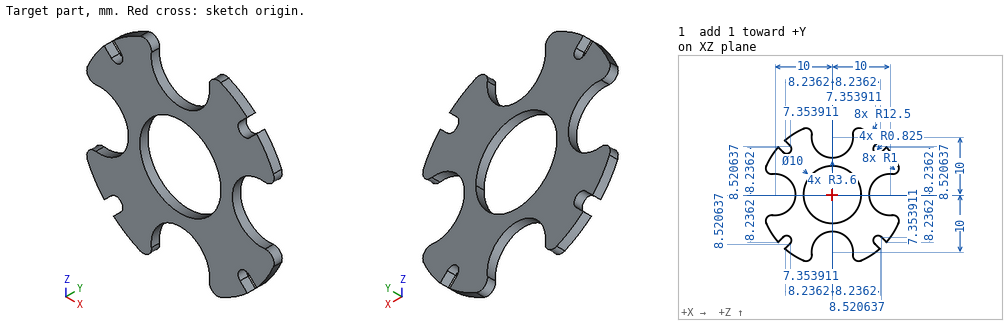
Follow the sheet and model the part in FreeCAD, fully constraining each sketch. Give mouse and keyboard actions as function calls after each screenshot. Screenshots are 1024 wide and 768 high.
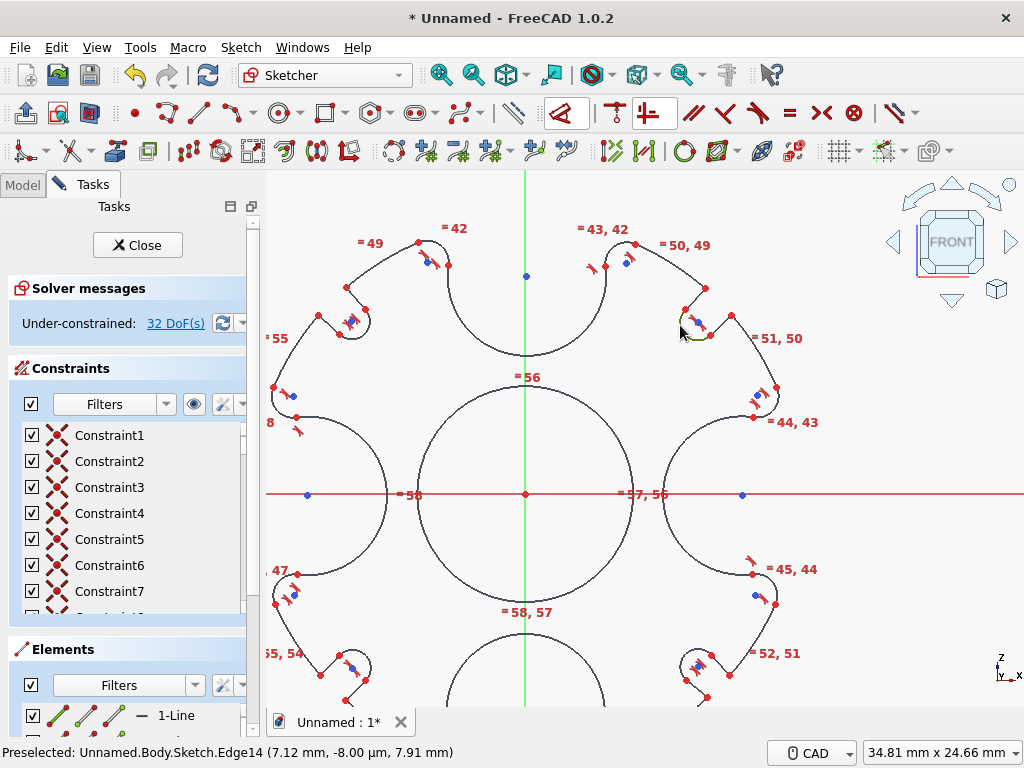
click(696, 649)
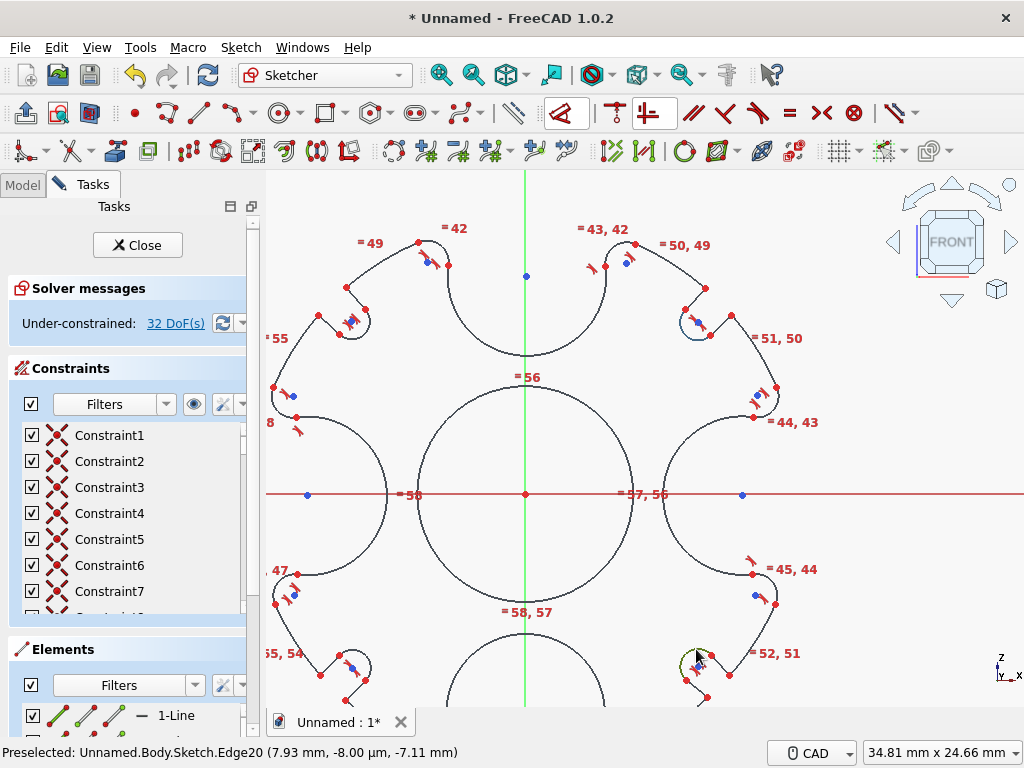
click(371, 665)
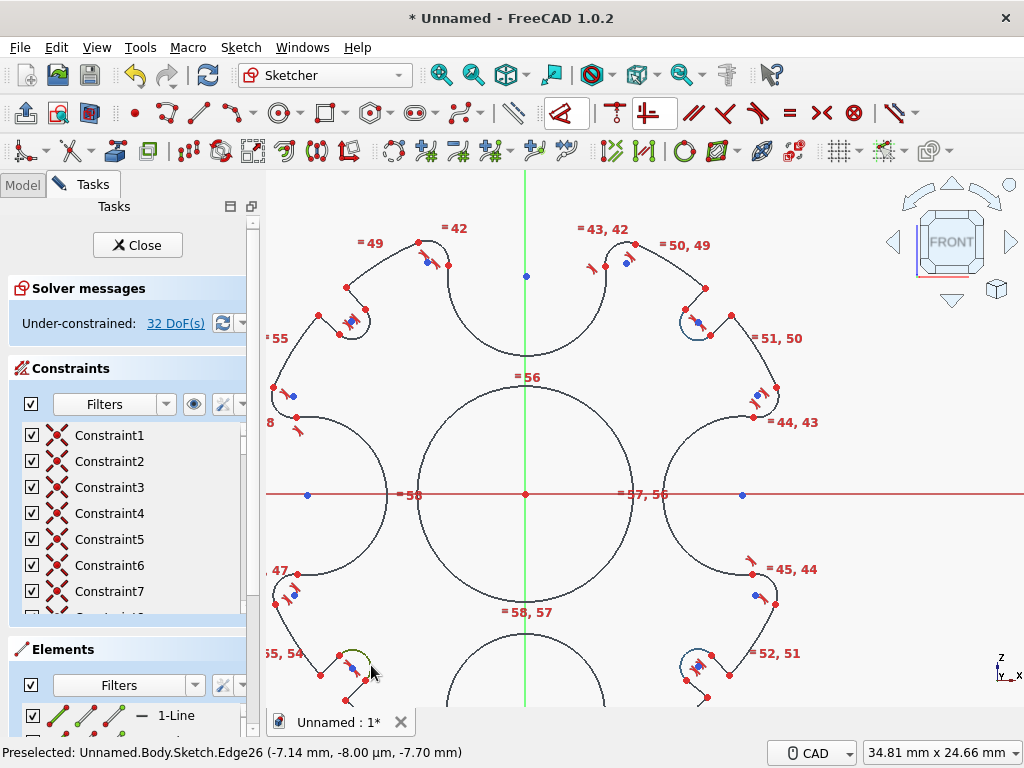
click(355, 339)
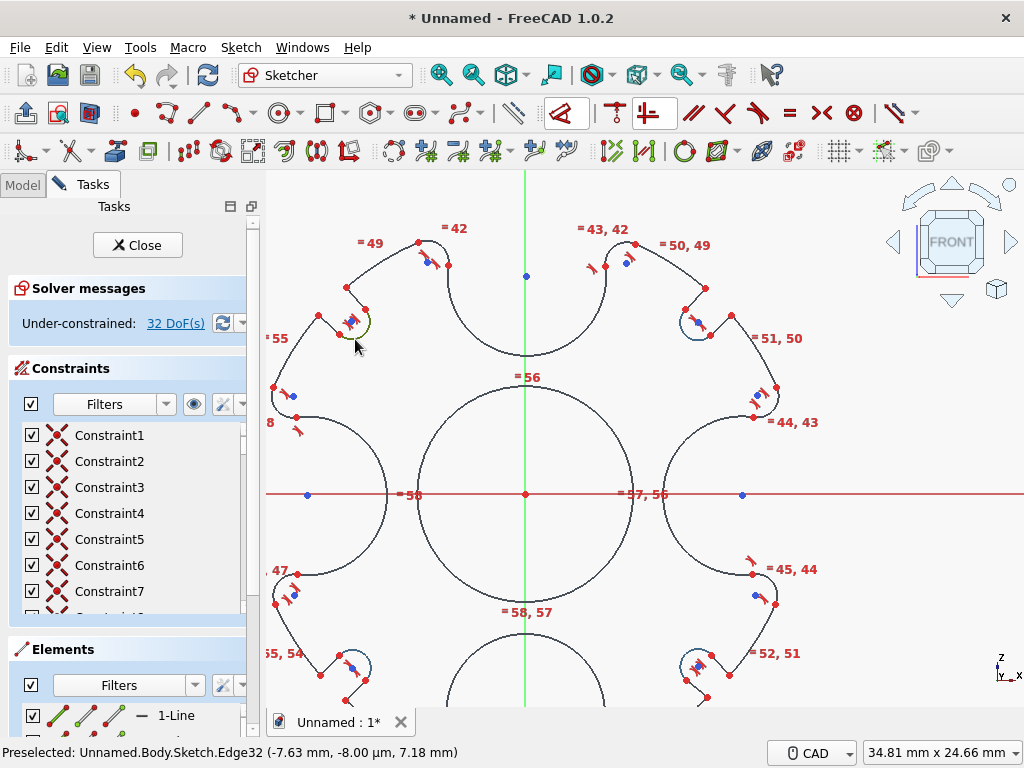
click(790, 114)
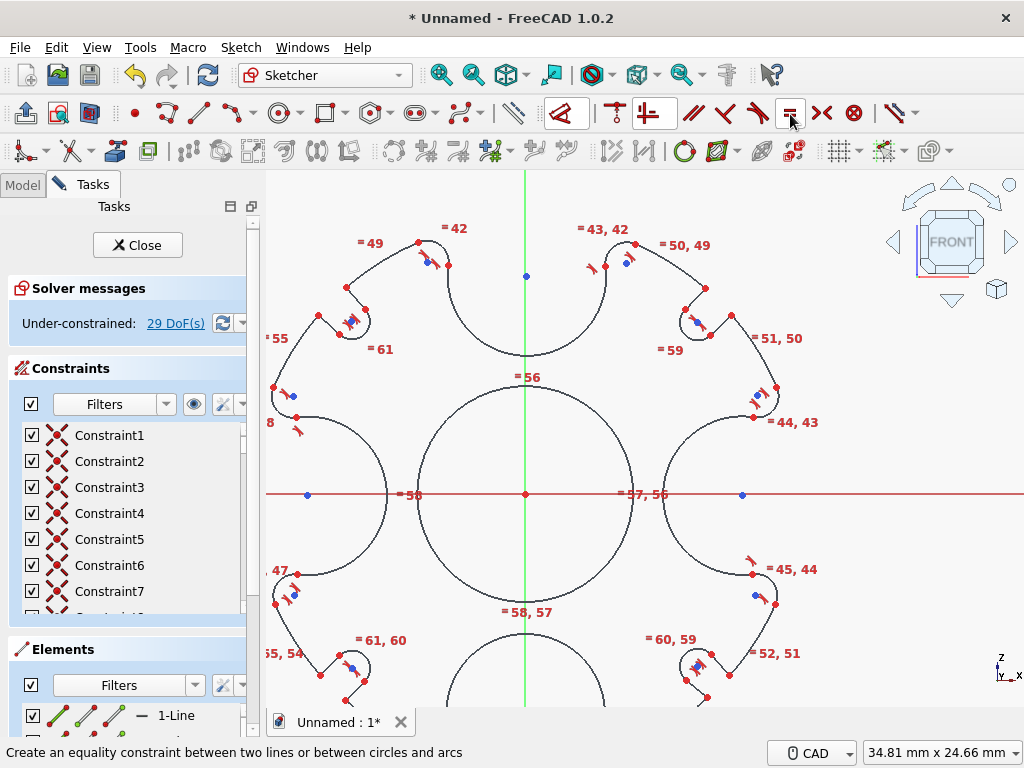
click(527, 277)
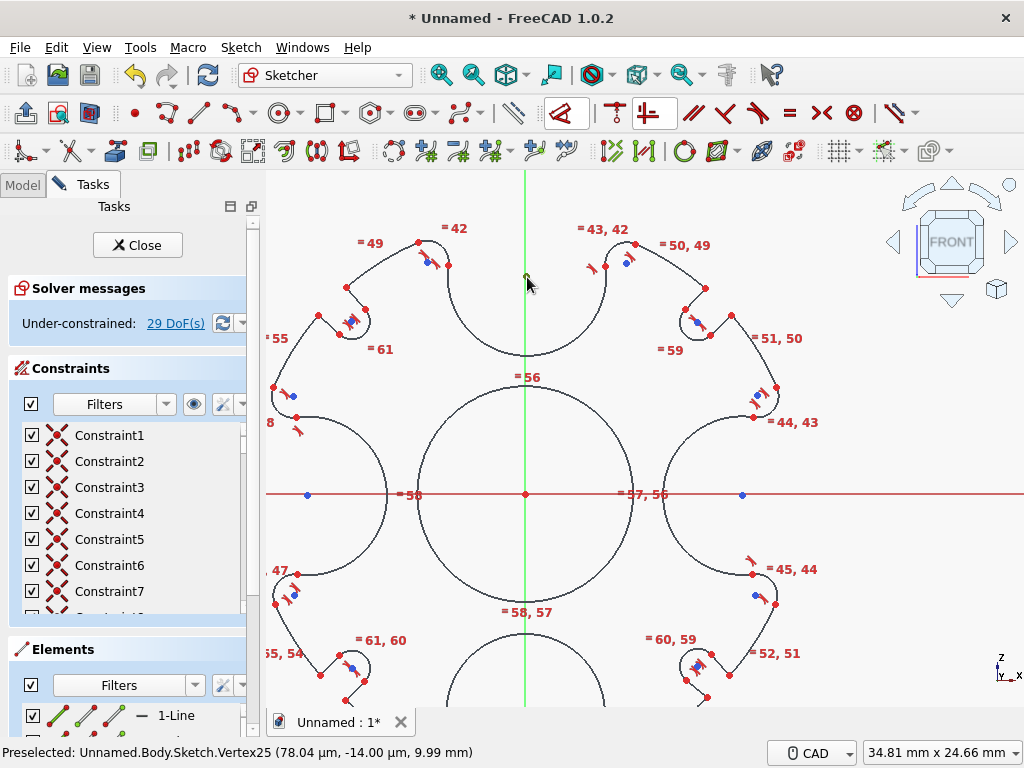
click(525, 542)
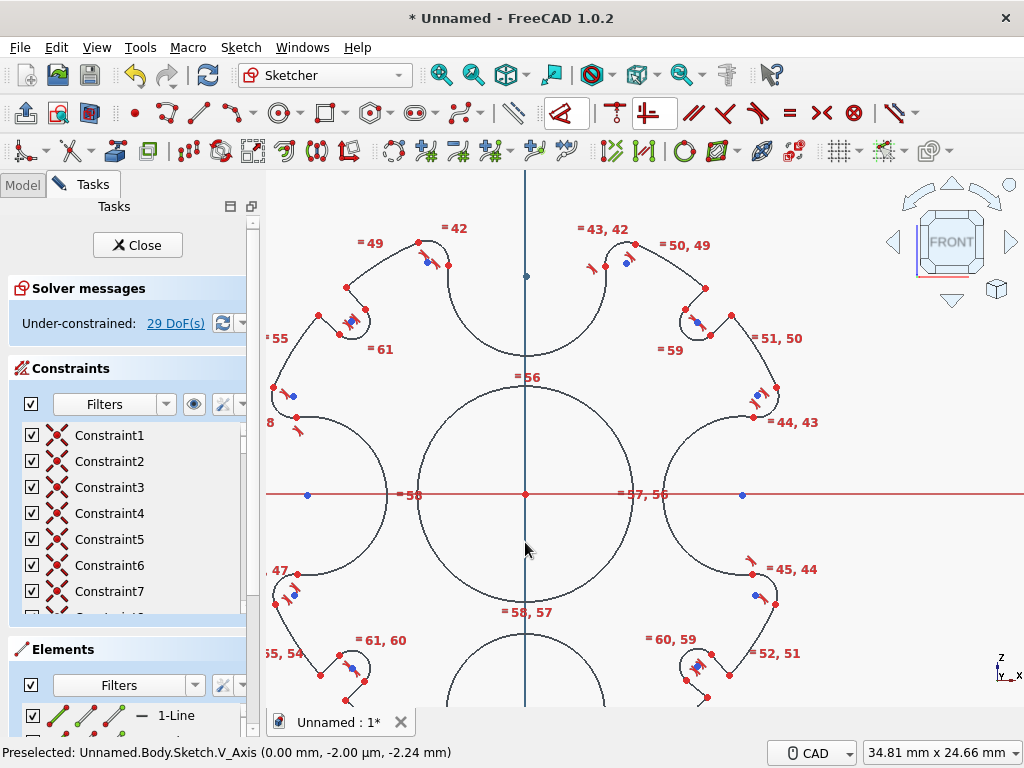
click(616, 114)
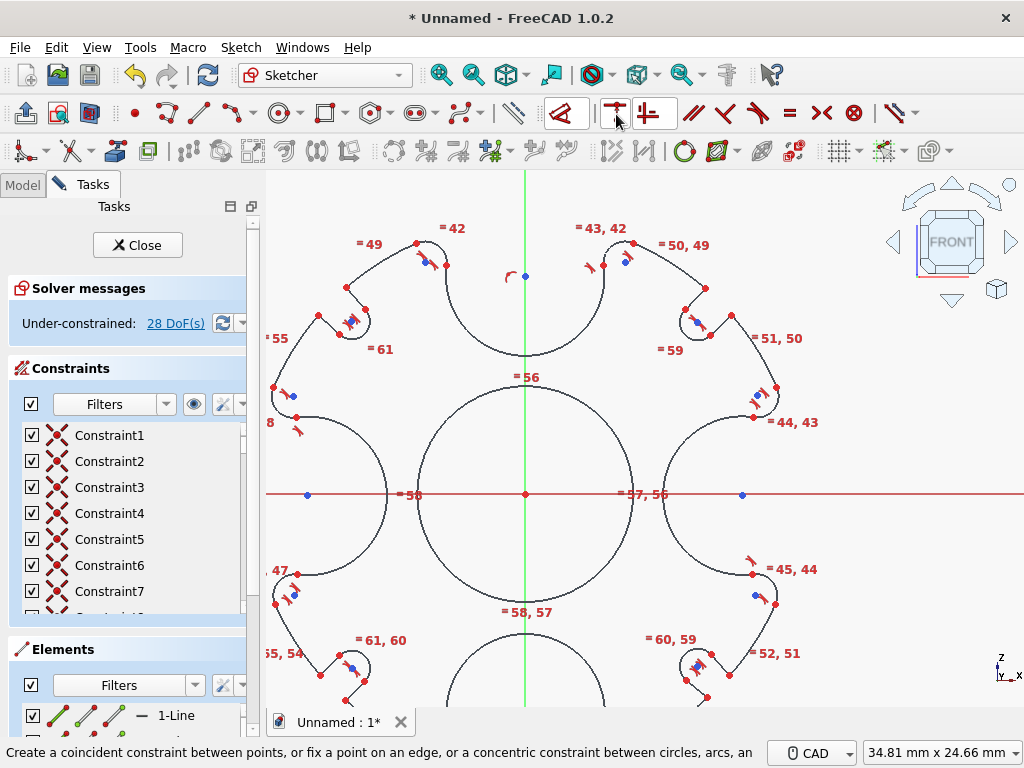
click(742, 496)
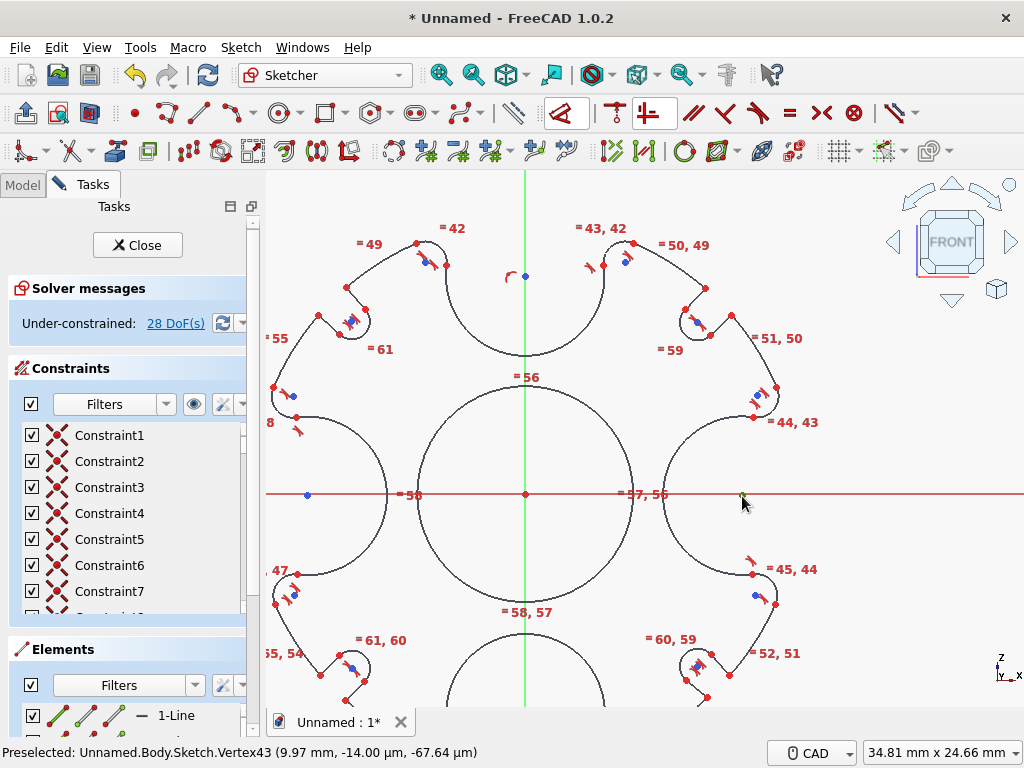
click(334, 494)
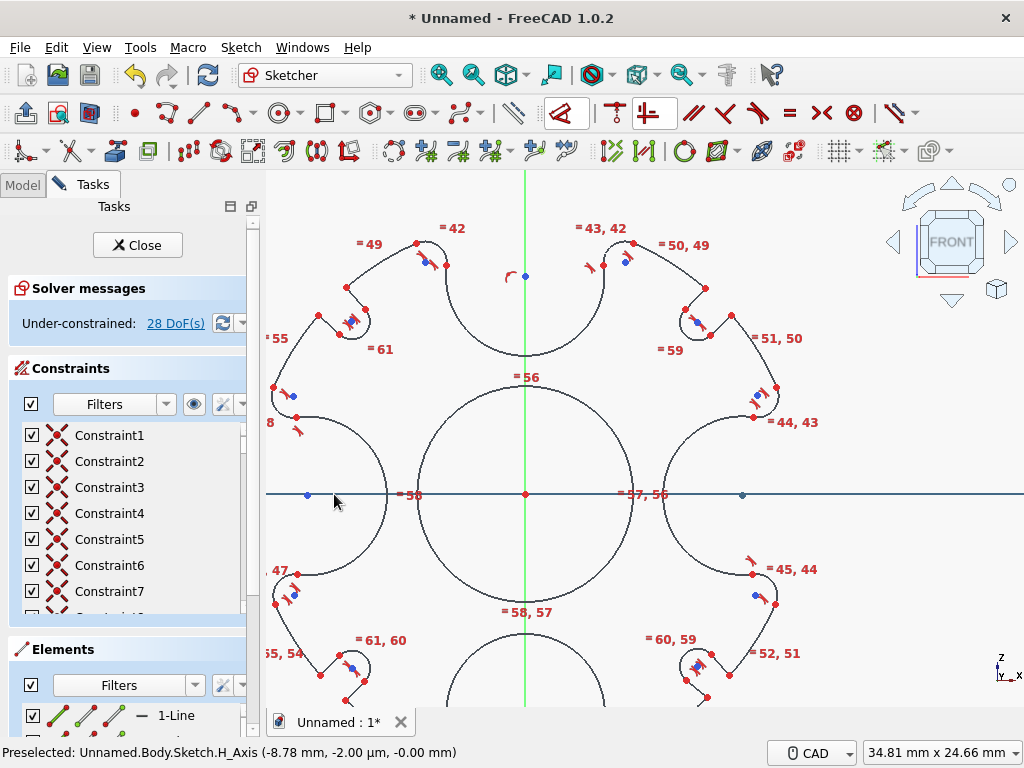
key(c)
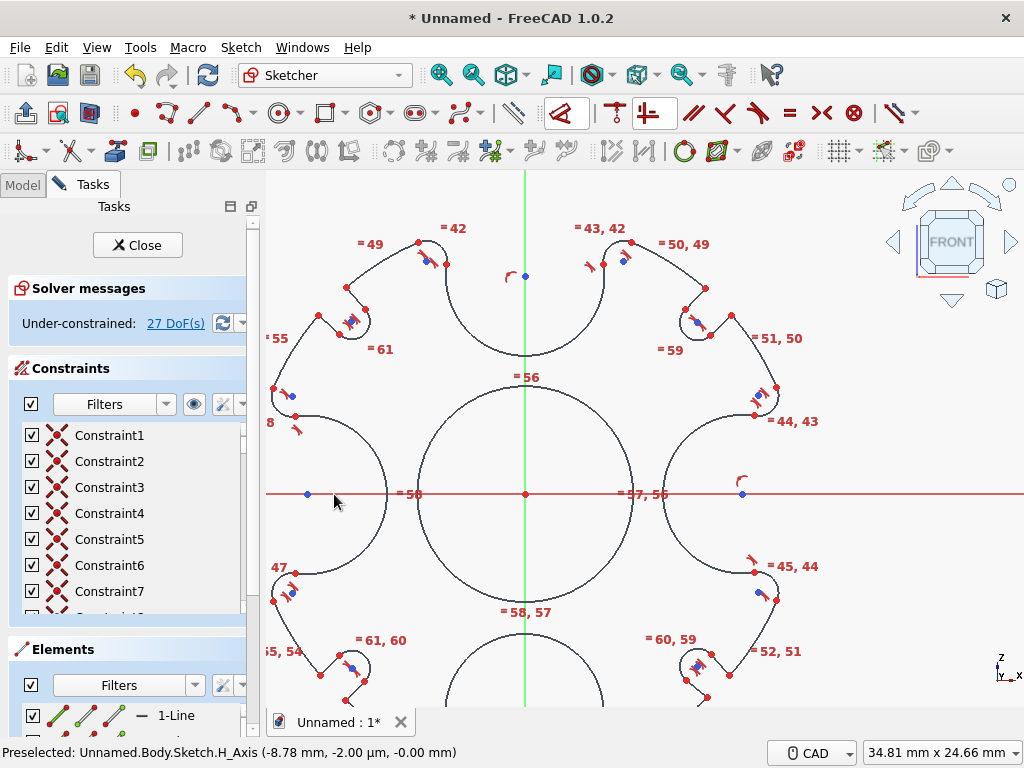
scroll(681, 325, down, 2)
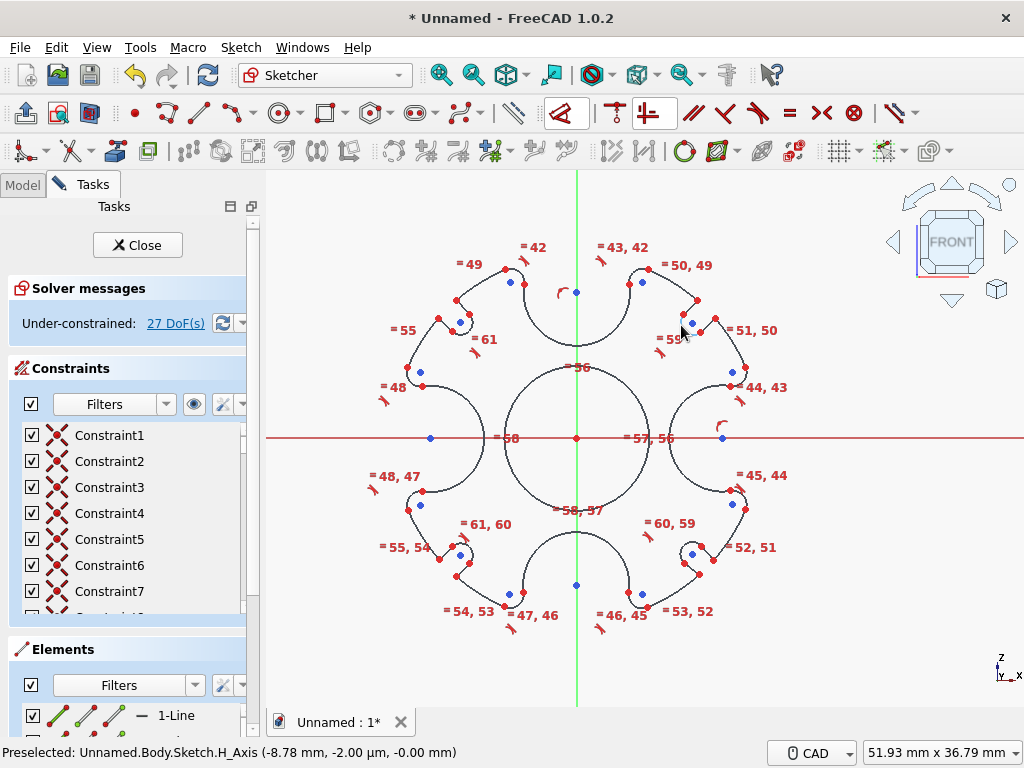
click(576, 585)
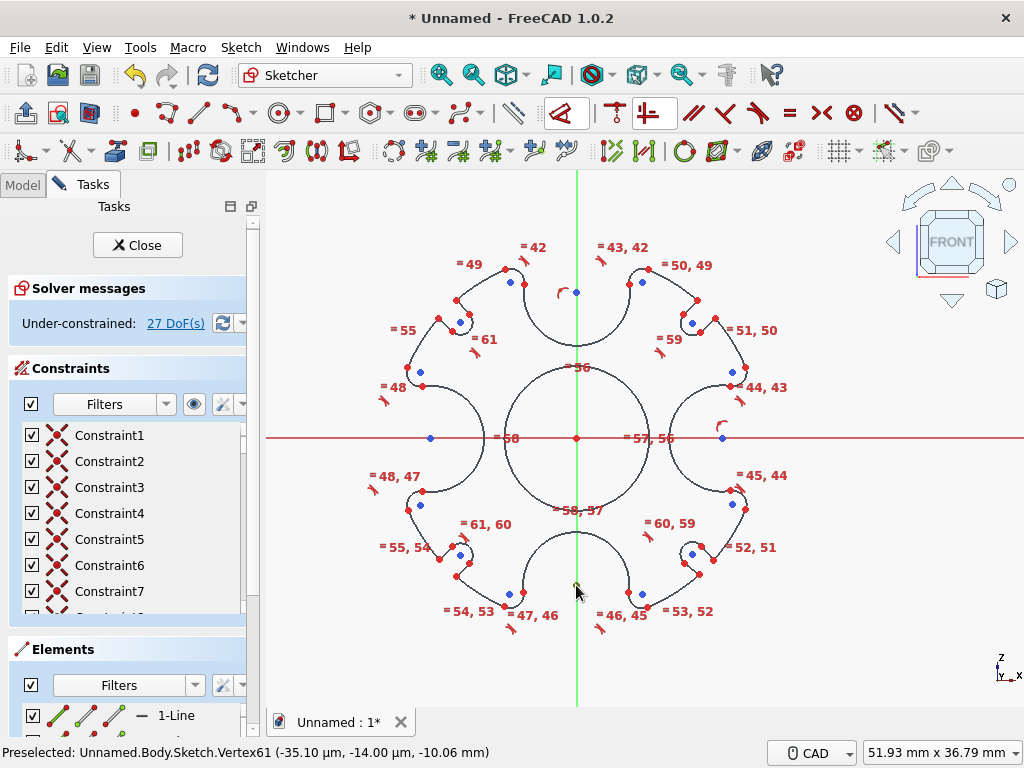
click(577, 645)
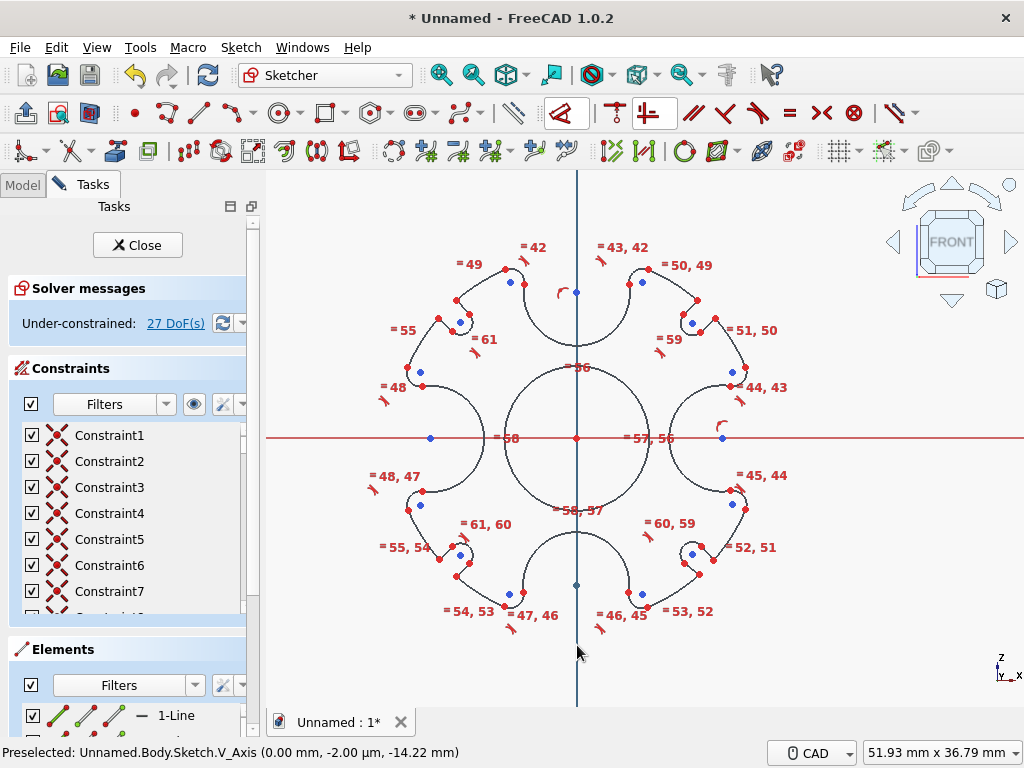
click(616, 114)